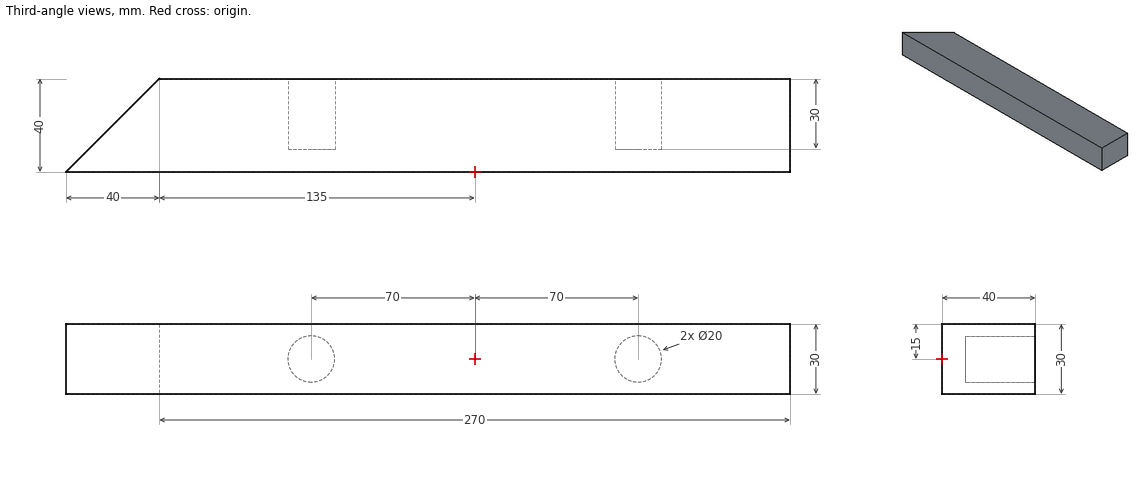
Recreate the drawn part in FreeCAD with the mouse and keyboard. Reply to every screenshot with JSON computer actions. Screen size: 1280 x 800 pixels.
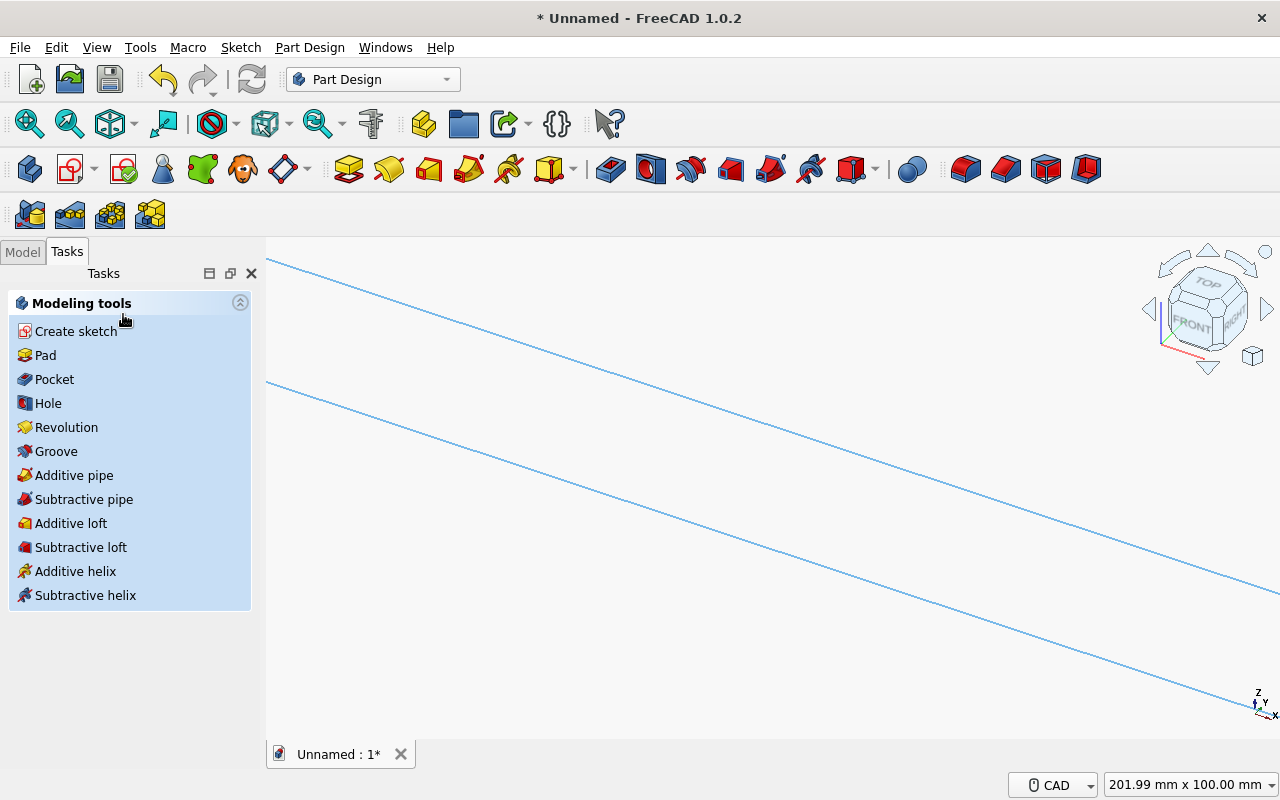
{"action": "left_click", "coordinate": [350, 170]}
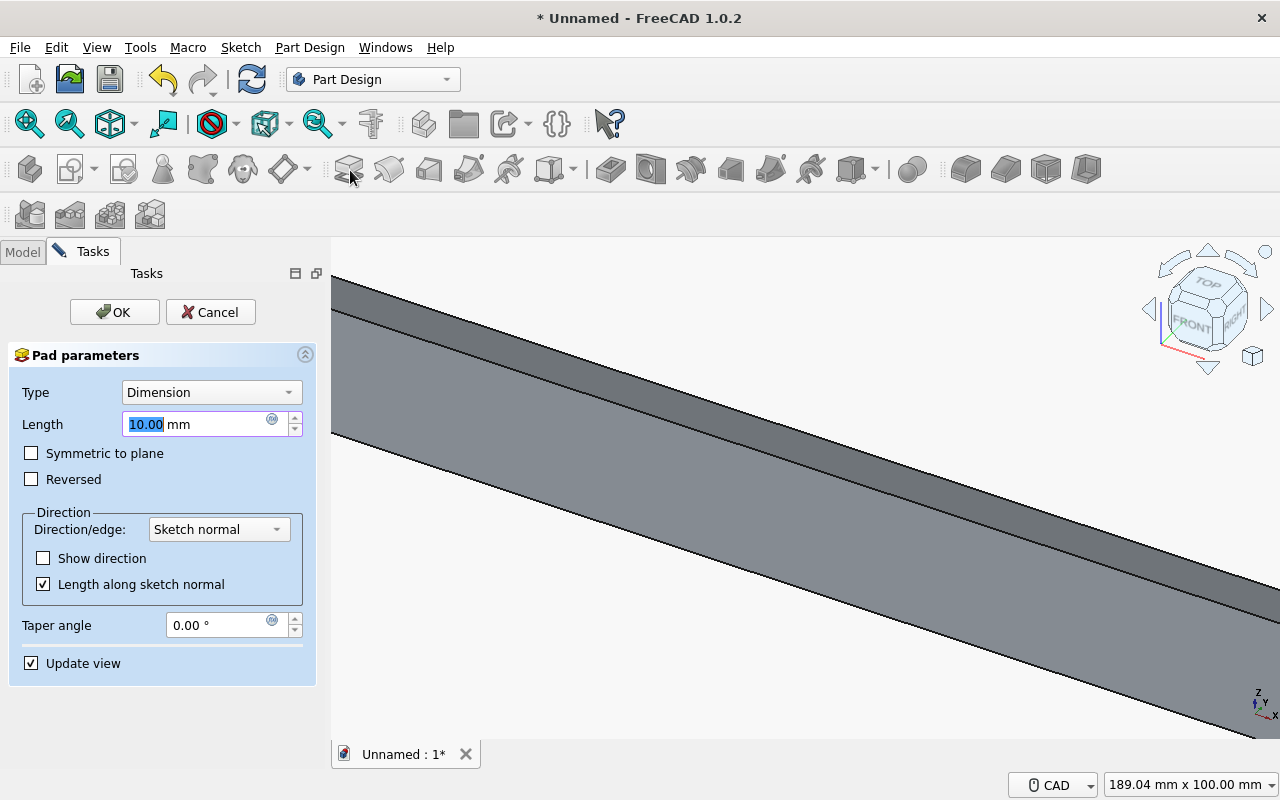
{"action": "type", "text": "40"}
{"action": "key", "text": "Tab"}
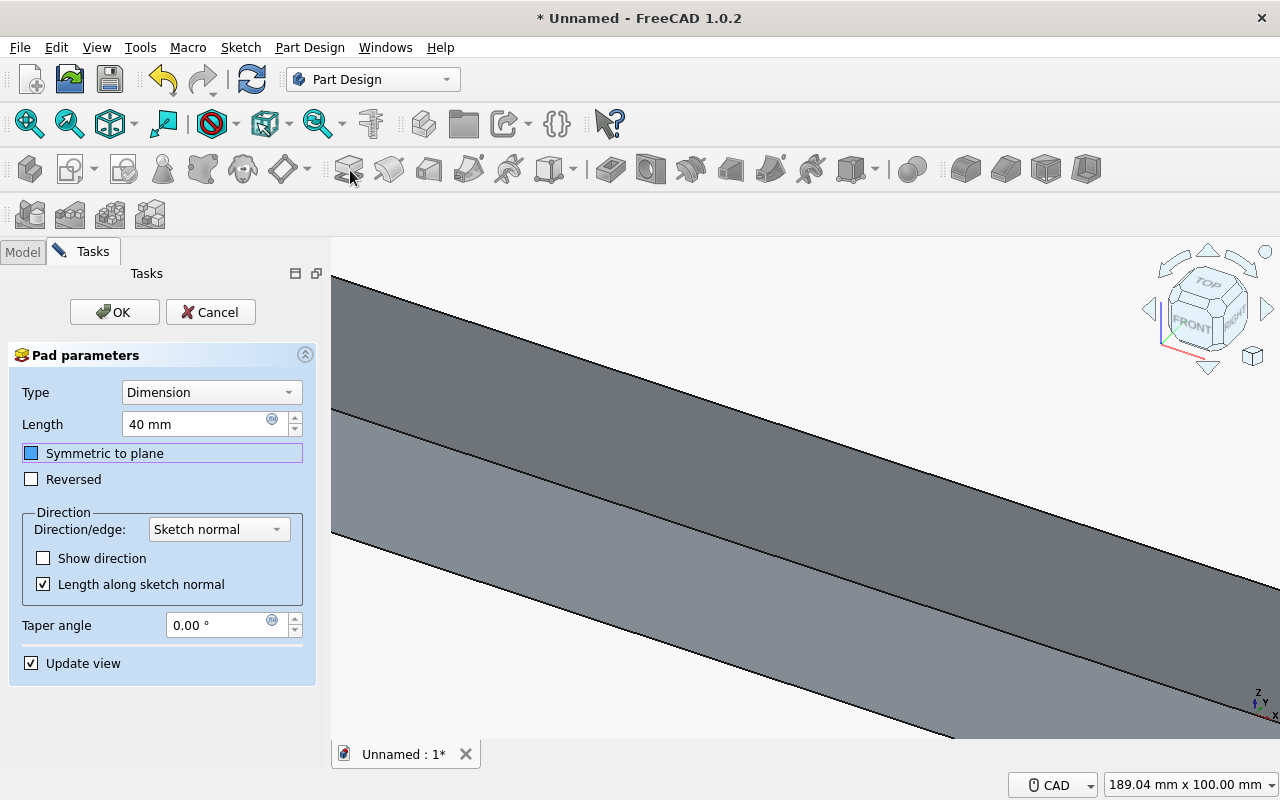
{"action": "left_click", "coordinate": [30, 479]}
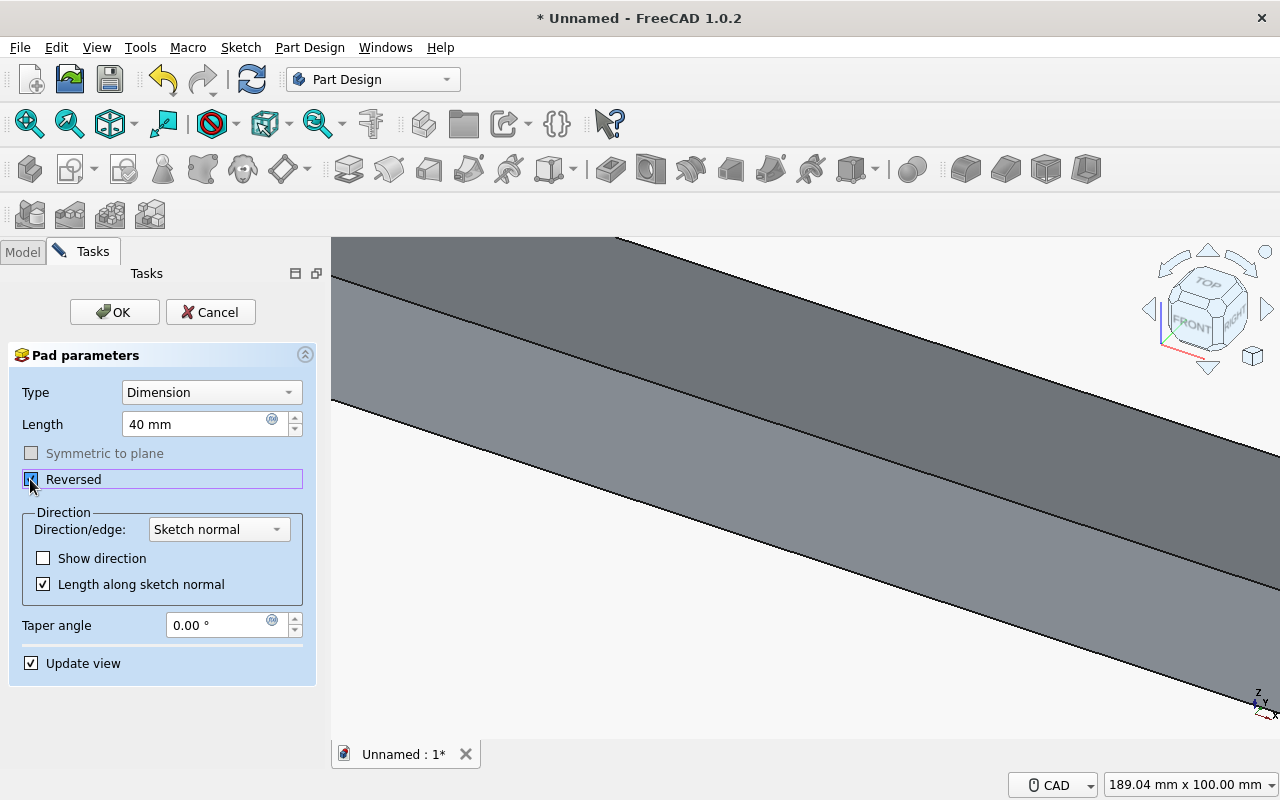
{"action": "left_click", "coordinate": [115, 312]}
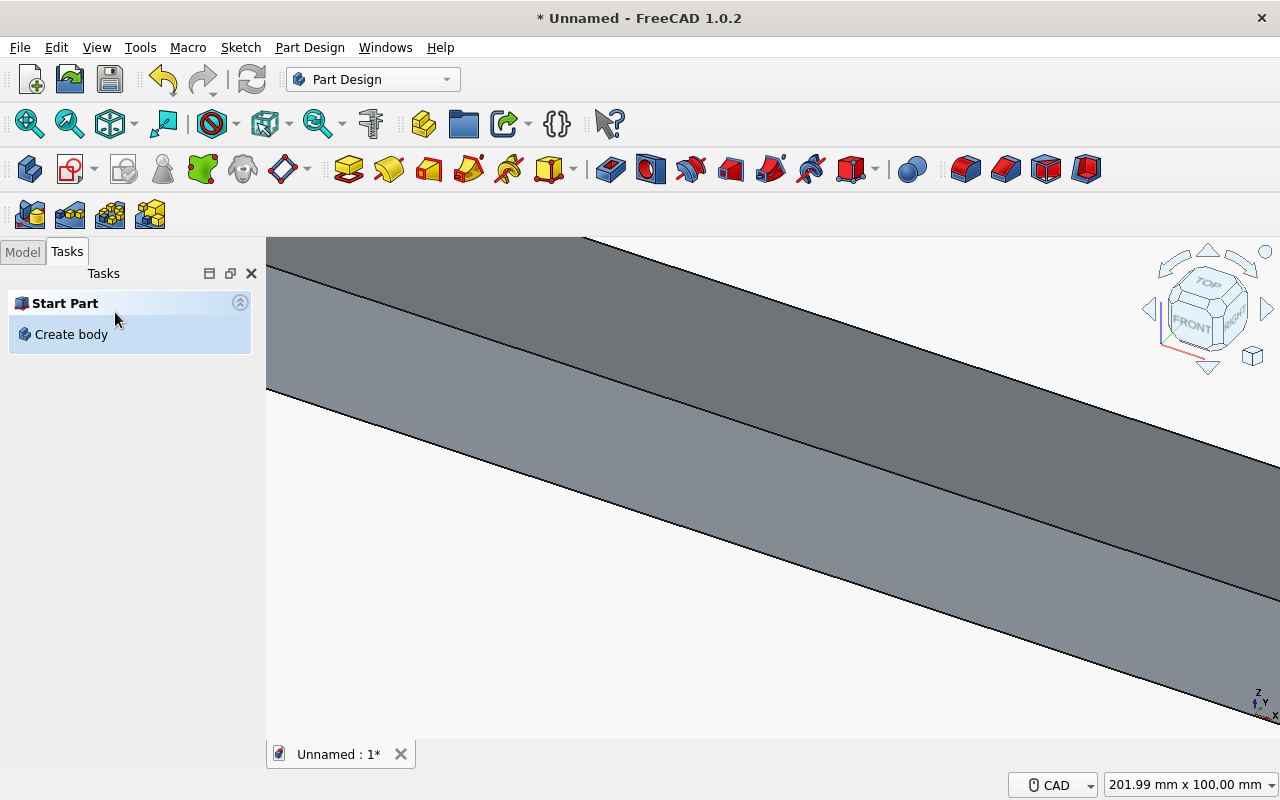
{"action": "left_click", "coordinate": [30, 124]}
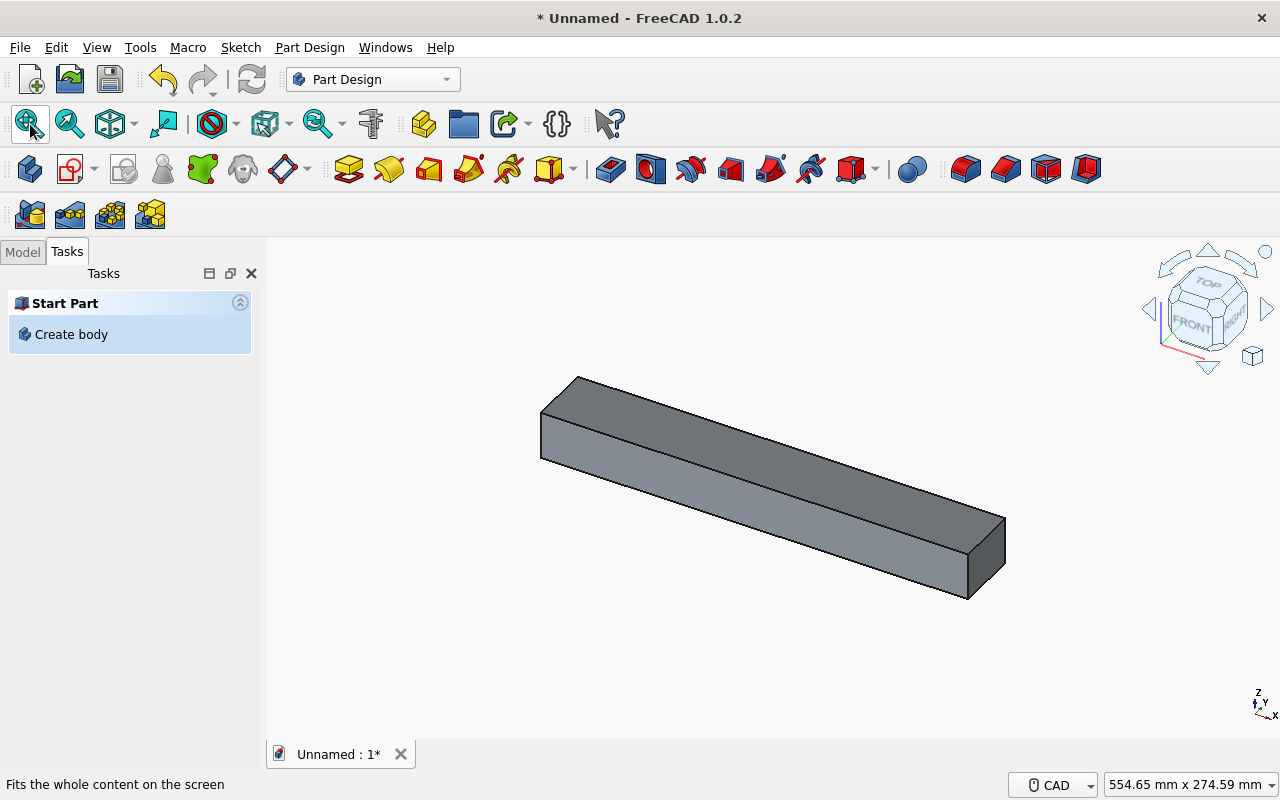
{"action": "key", "text": "4"}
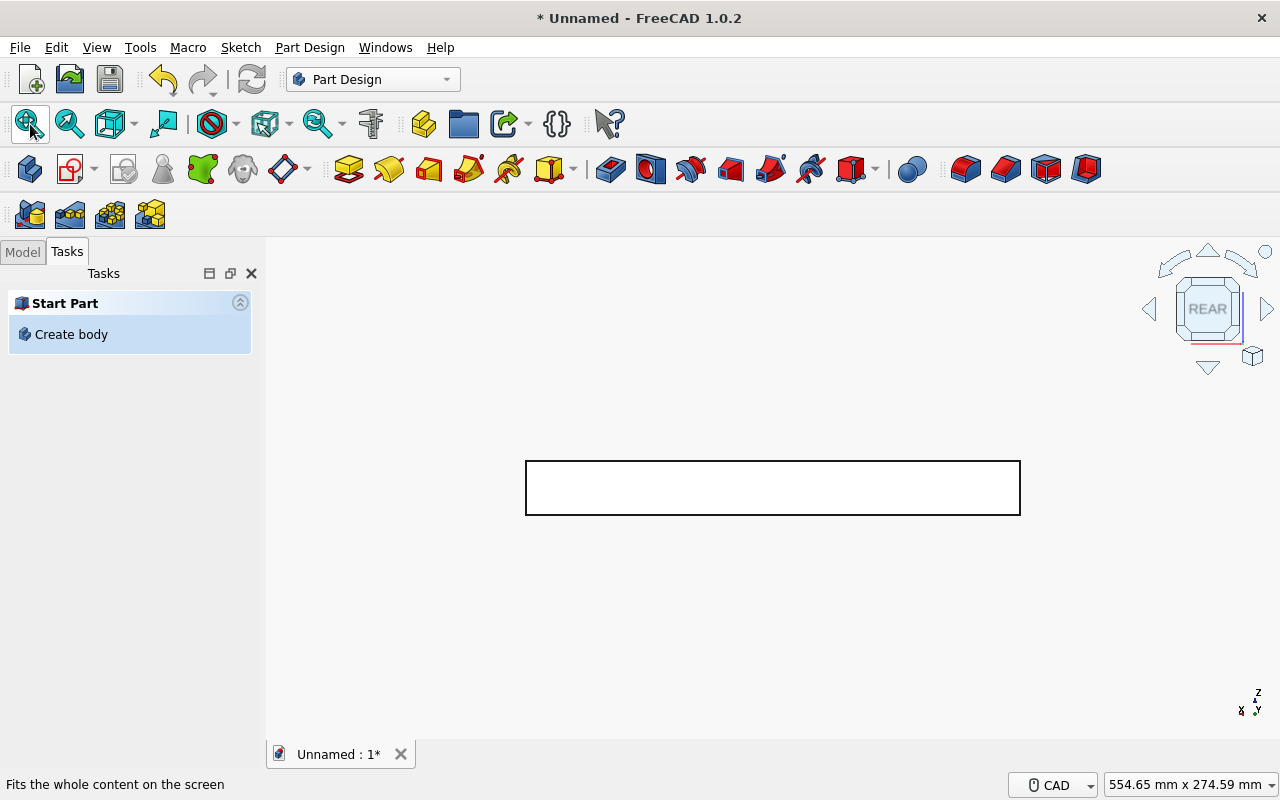
{"action": "left_click", "coordinate": [561, 487]}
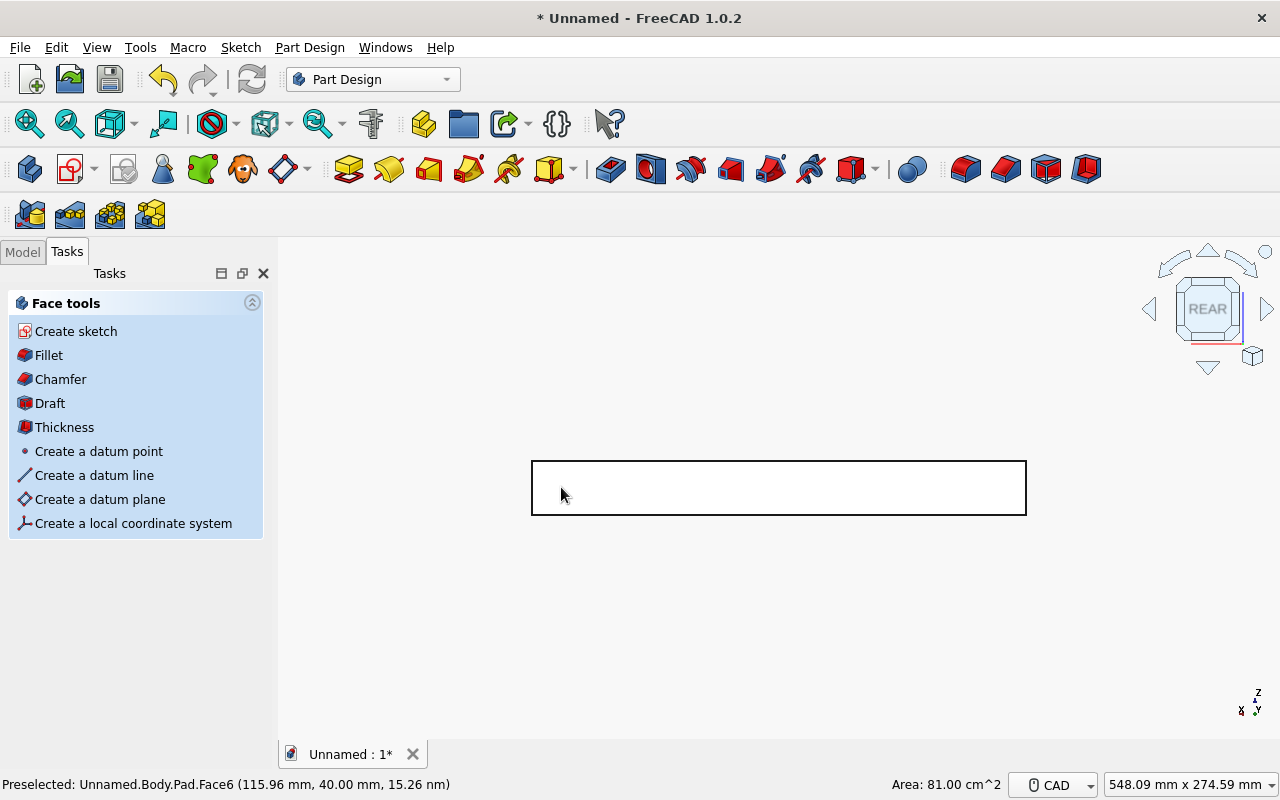
{"action": "left_click", "coordinate": [70, 170]}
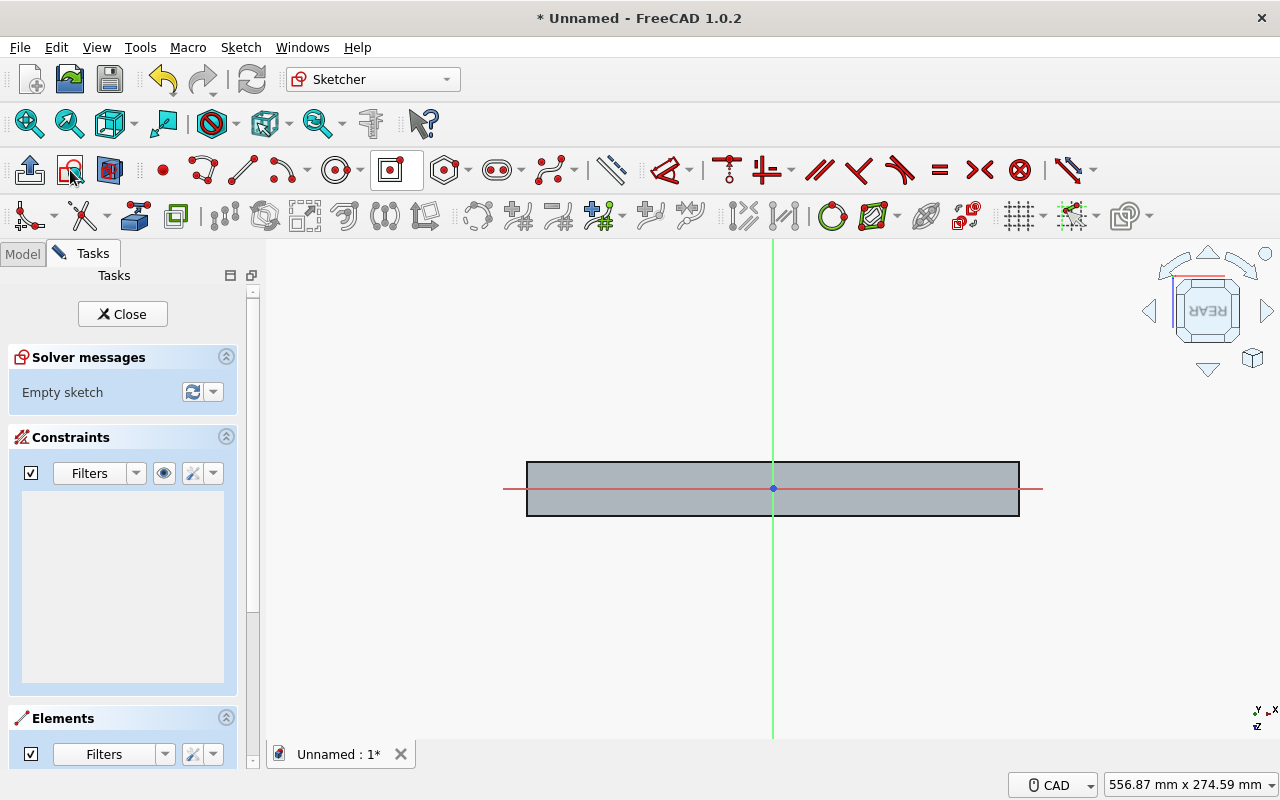
{"action": "scroll", "coordinate": [856, 489], "scroll_direction": "up", "scroll_amount": 3}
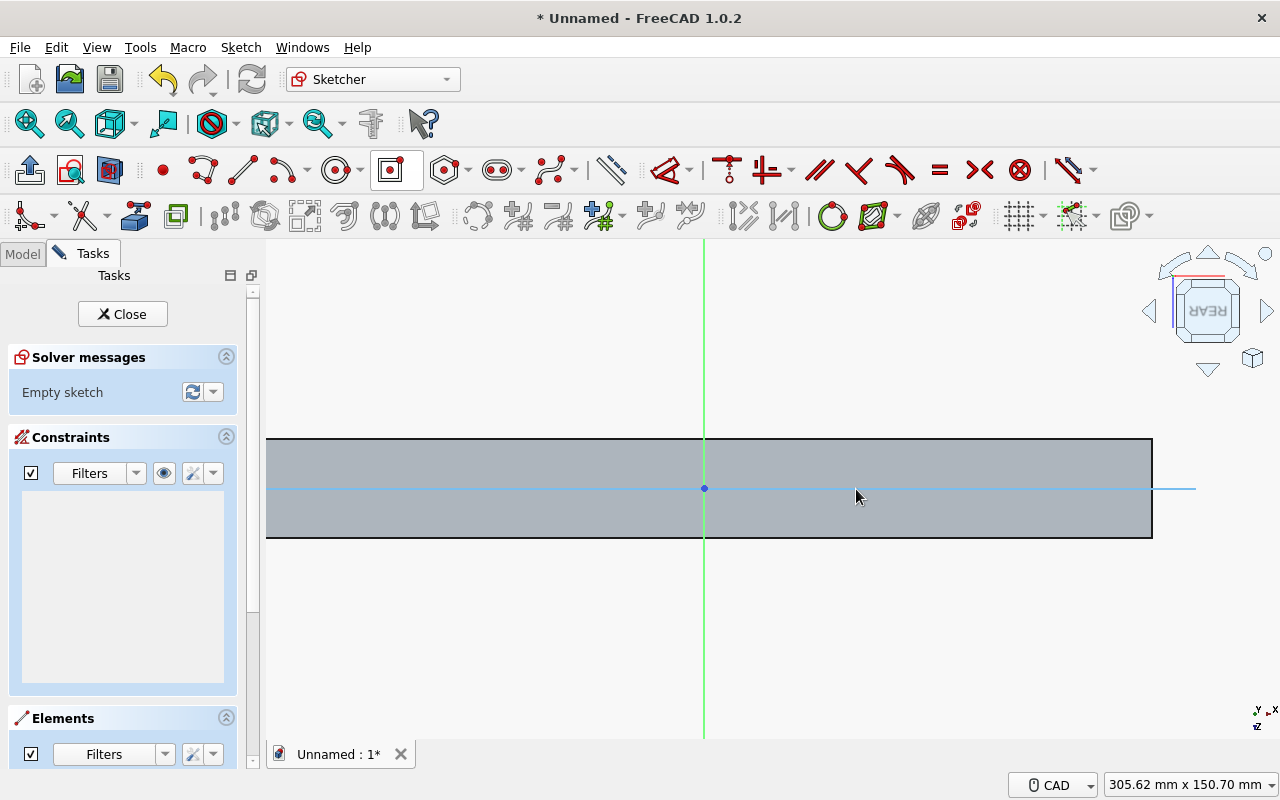
{"action": "left_click", "coordinate": [336, 170]}